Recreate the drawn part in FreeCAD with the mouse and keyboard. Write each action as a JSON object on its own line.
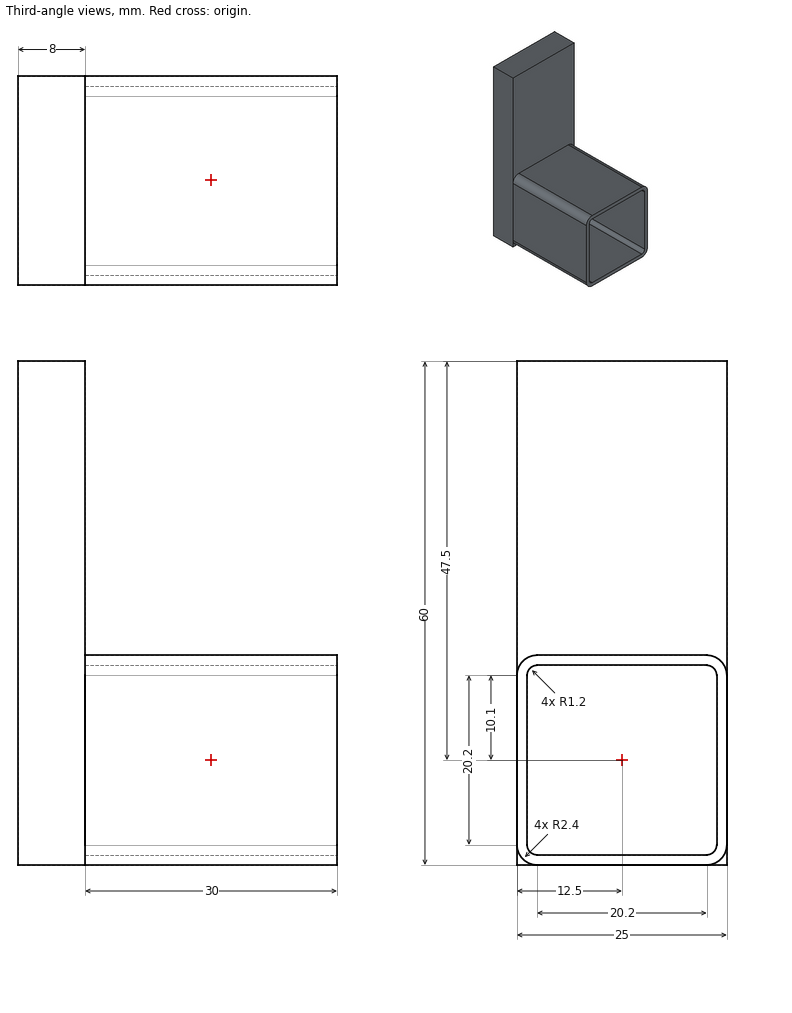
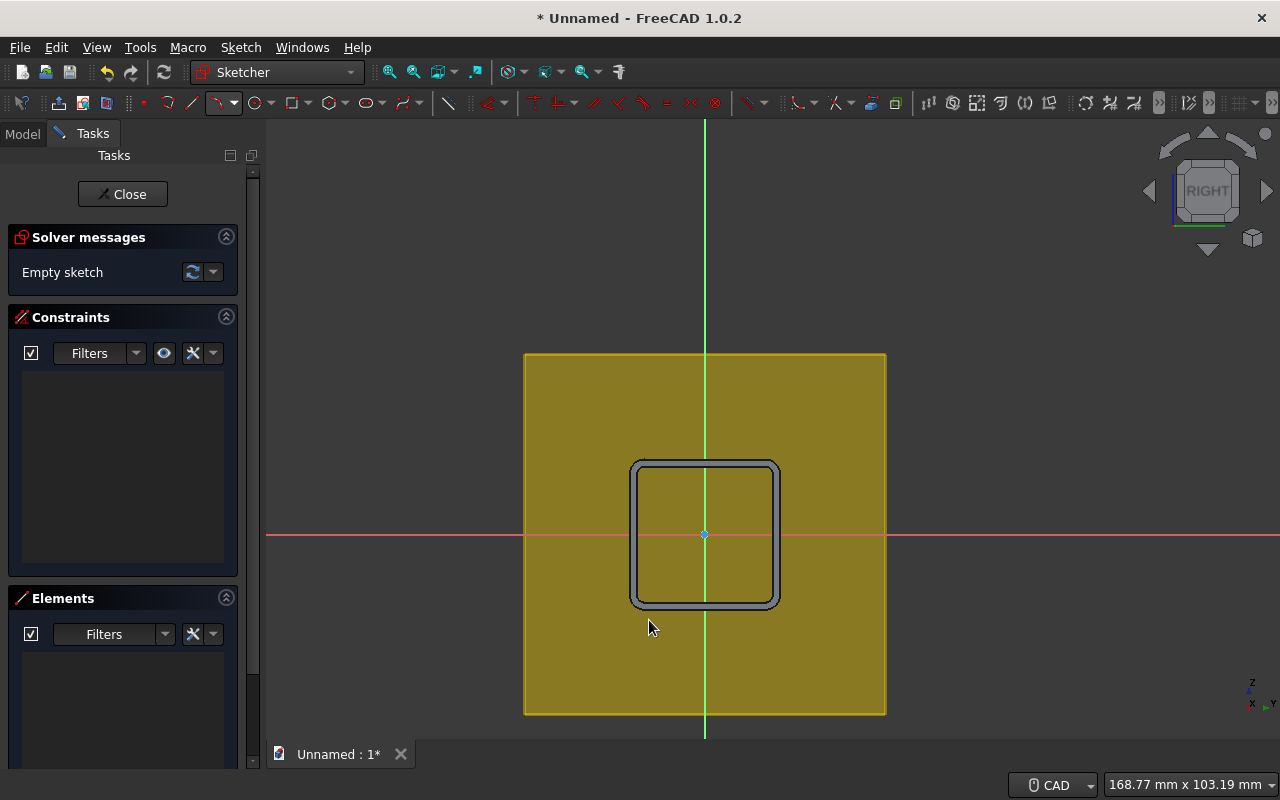
{"action": "left_click", "coordinate": [292, 104]}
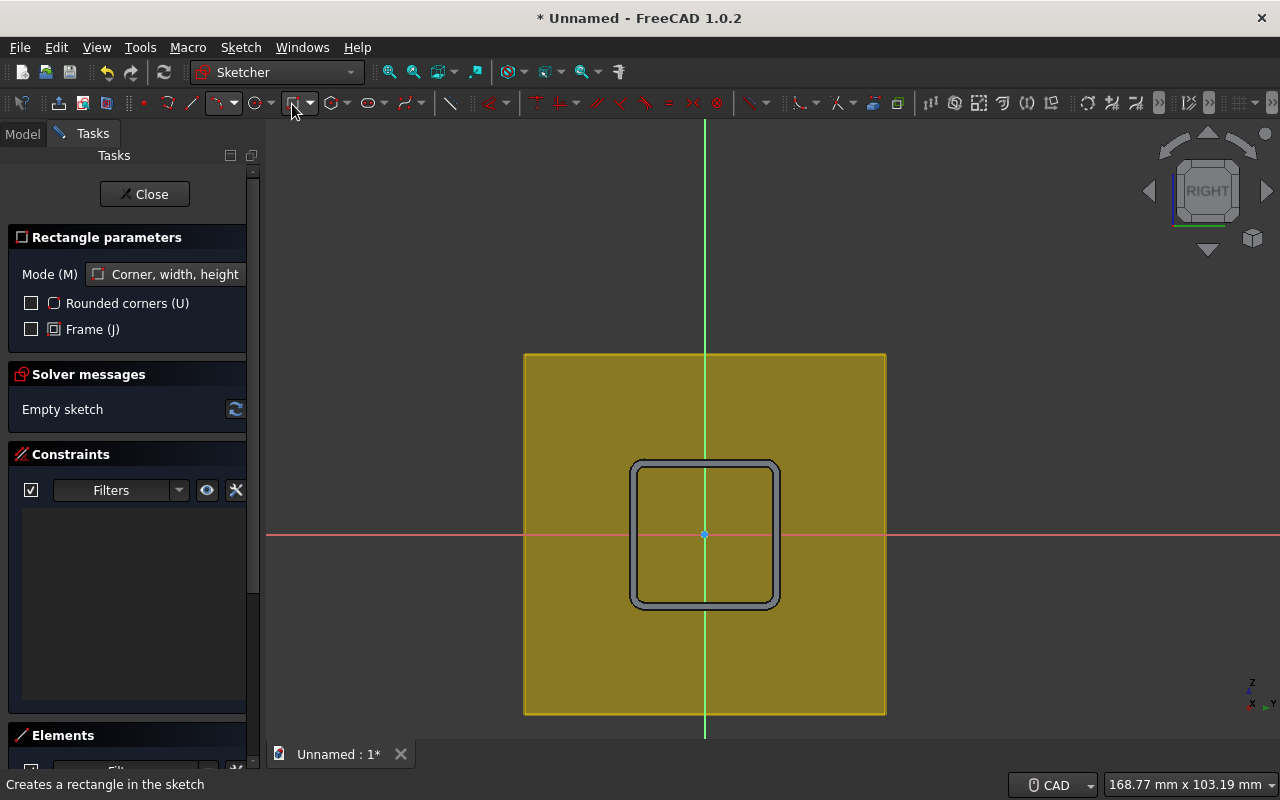
{"action": "left_click", "coordinate": [630, 249]}
{"action": "left_click", "coordinate": [780, 610]}
{"action": "key", "text": "Escape"}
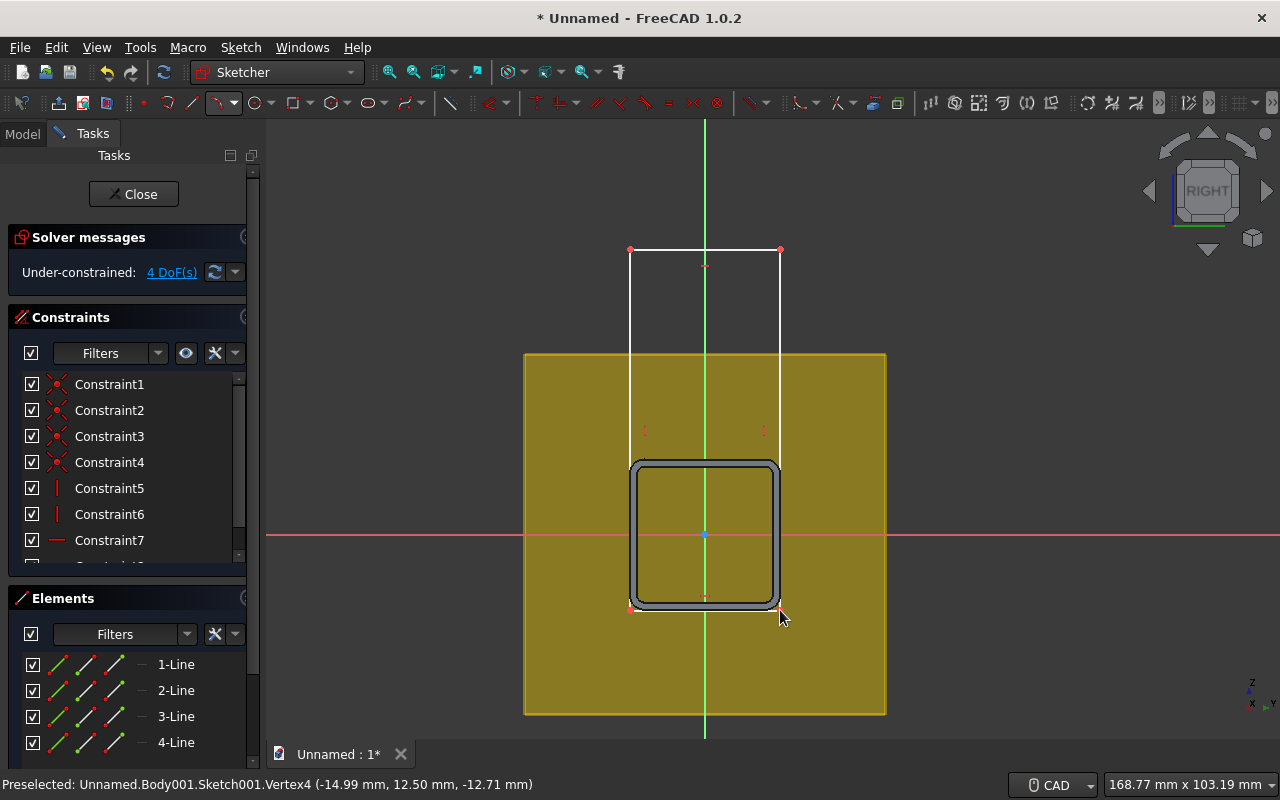
{"action": "key", "text": "d"}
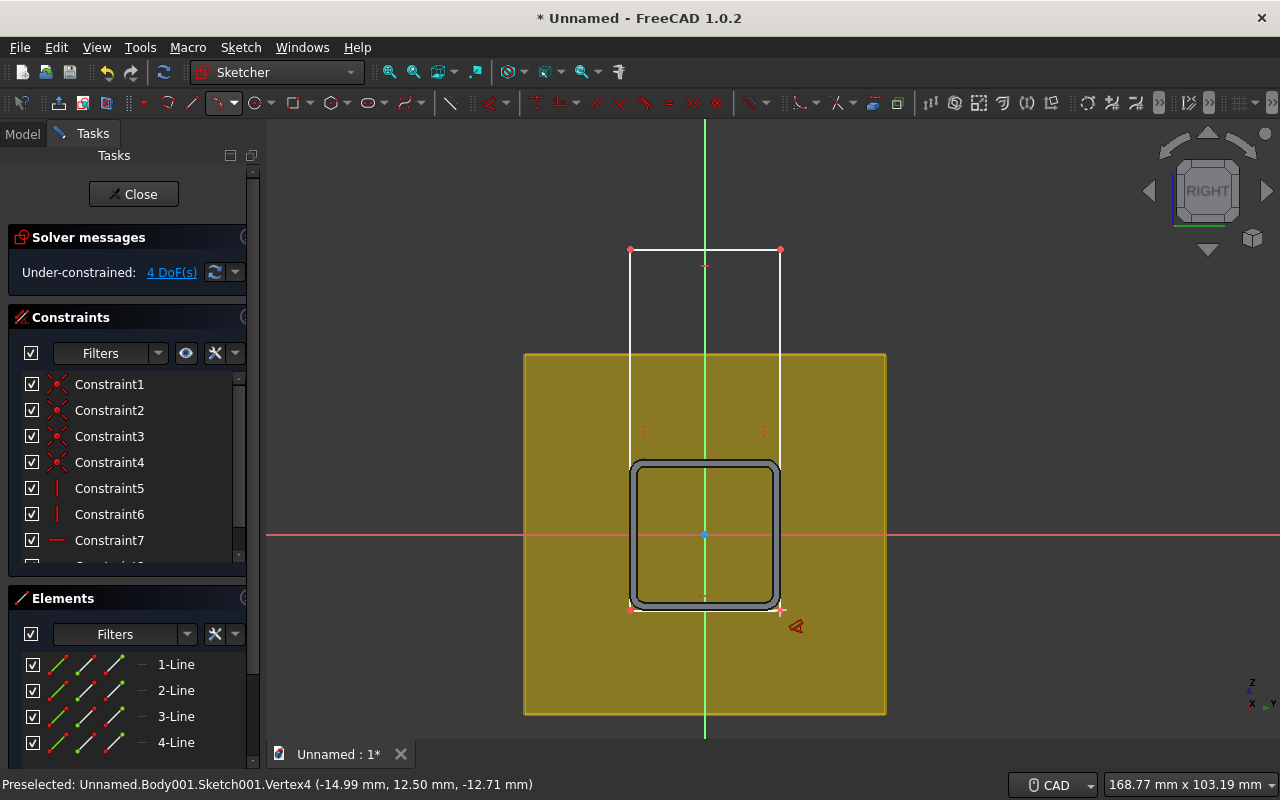
{"action": "left_click", "coordinate": [630, 358]}
{"action": "left_click", "coordinate": [596, 430]}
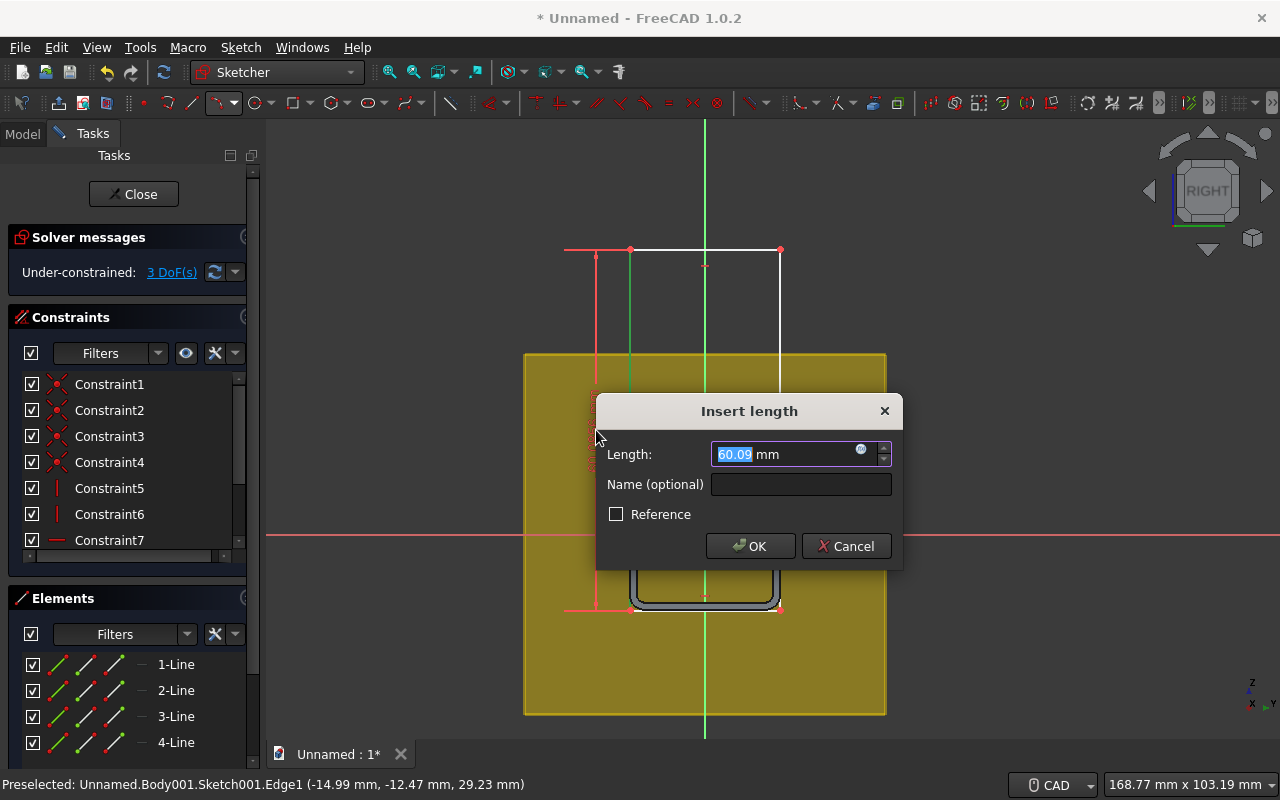
{"action": "type", "text": "60"}
{"action": "key", "text": "Return"}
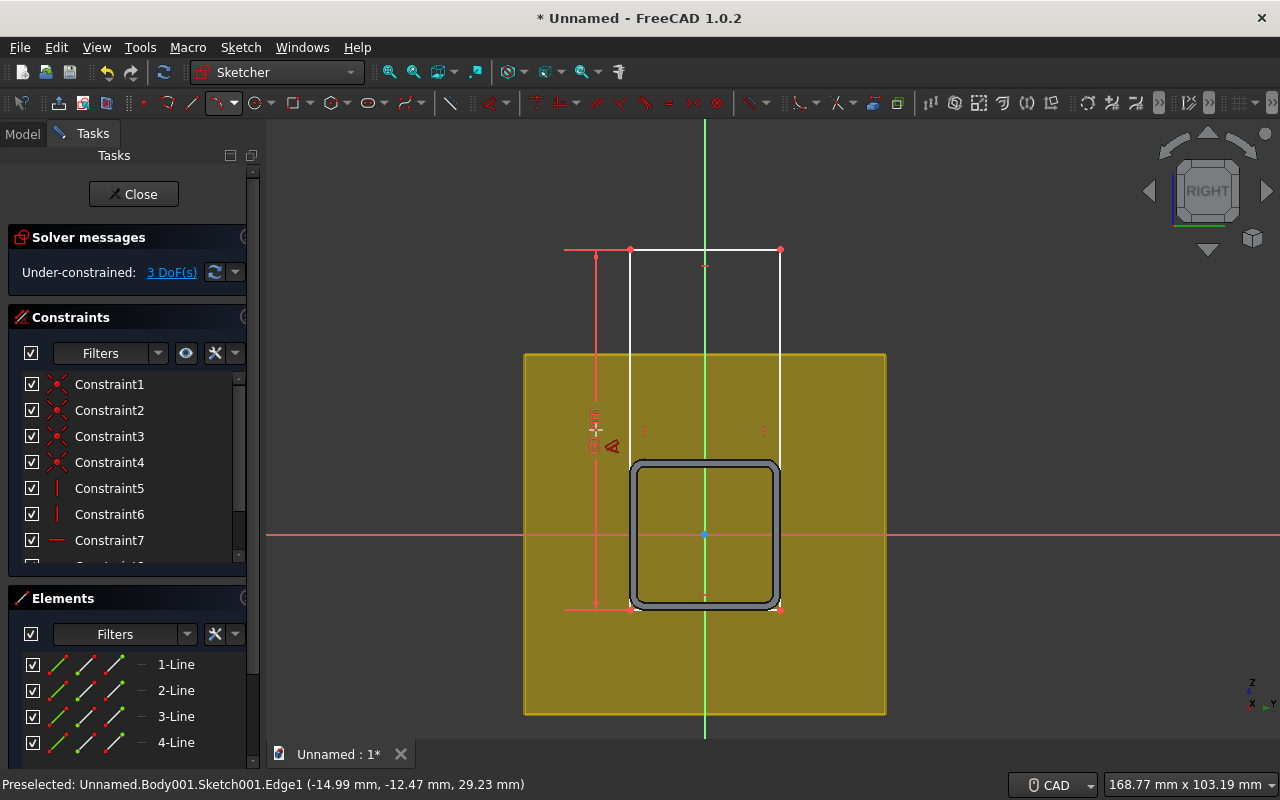
{"action": "left_click", "coordinate": [675, 610]}
{"action": "left_click", "coordinate": [671, 644]}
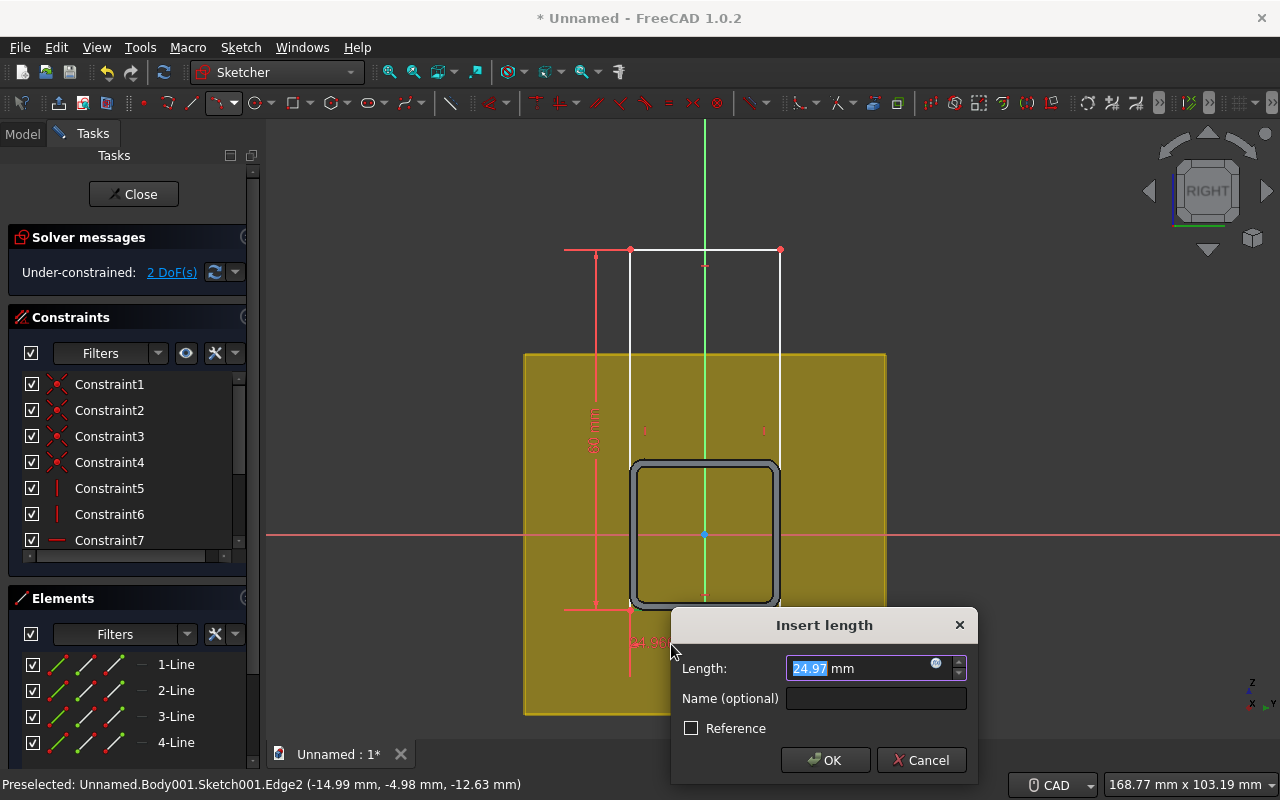
{"action": "type", "text": "25"}
{"action": "key", "text": "Return"}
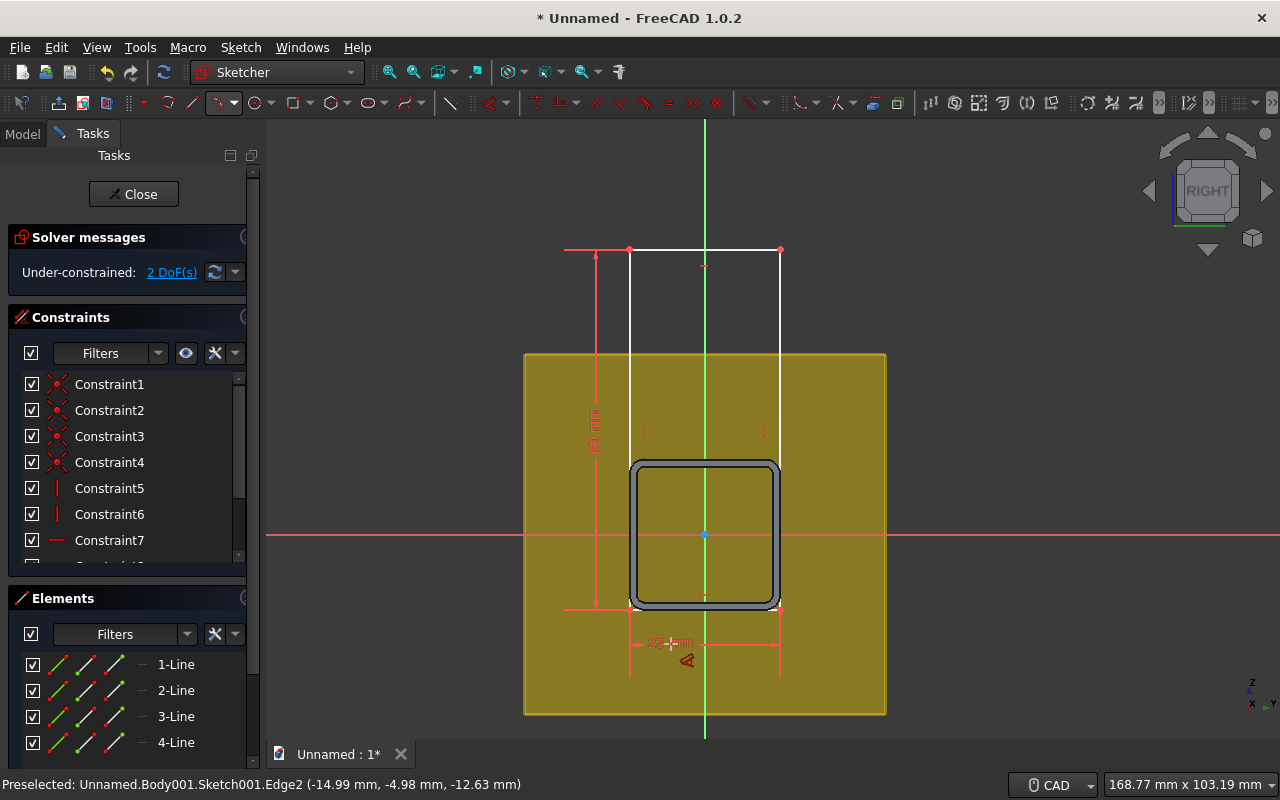
{"action": "left_click", "coordinate": [630, 250]}
{"action": "left_click", "coordinate": [667, 216]}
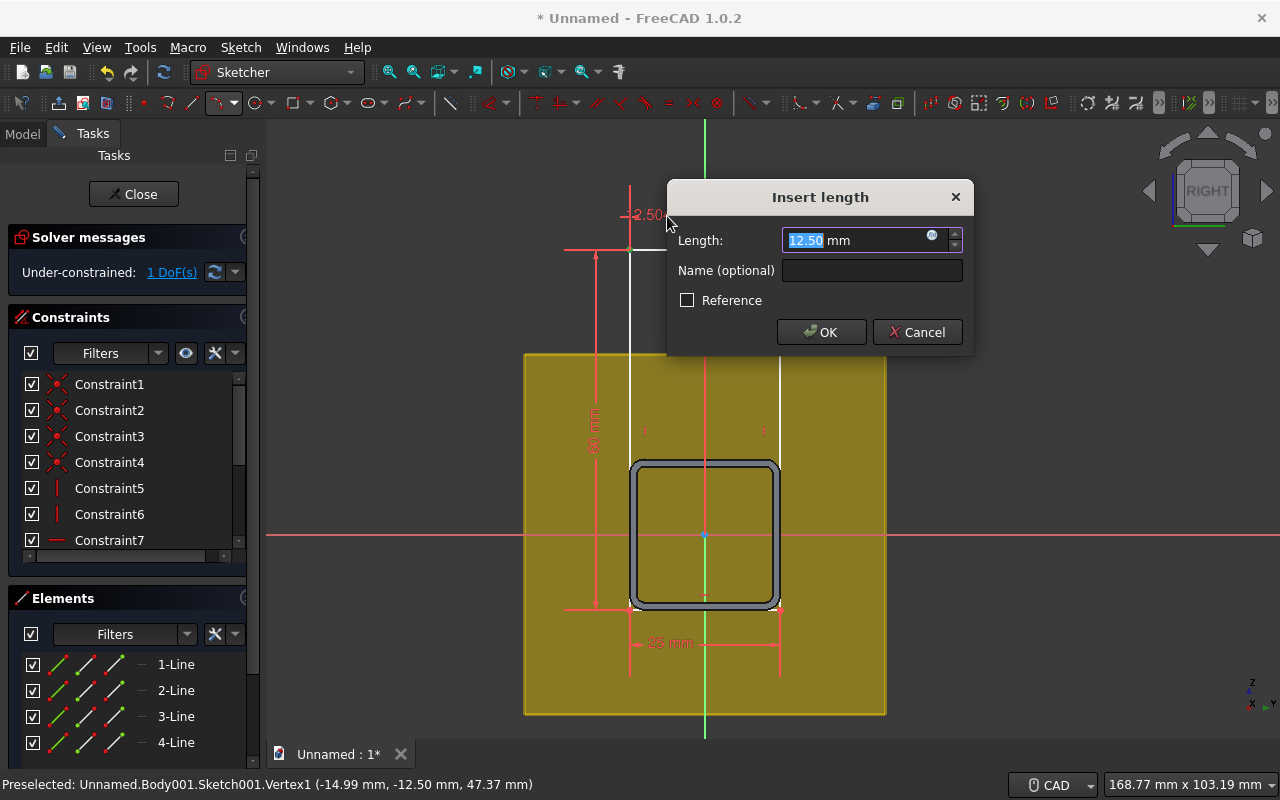
{"action": "type", "text": "12.5"}
{"action": "key", "text": "Return"}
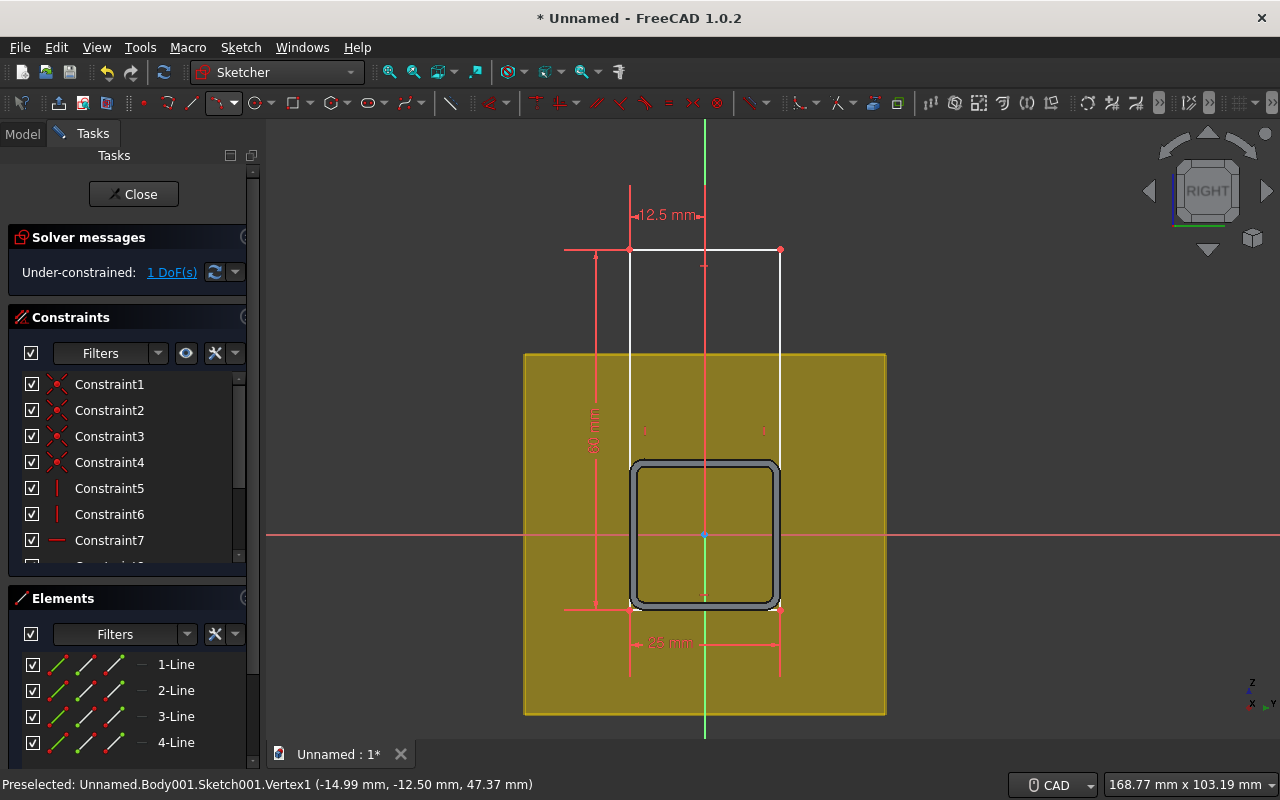
{"action": "left_click", "coordinate": [630, 250]}
{"action": "left_click", "coordinate": [596, 392]}